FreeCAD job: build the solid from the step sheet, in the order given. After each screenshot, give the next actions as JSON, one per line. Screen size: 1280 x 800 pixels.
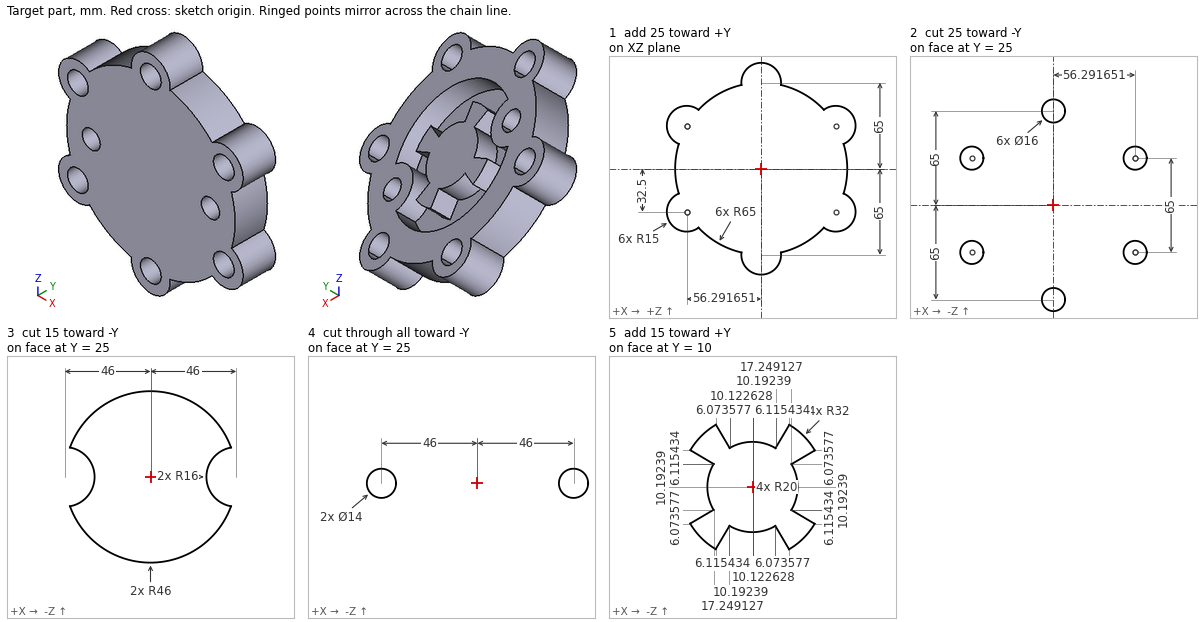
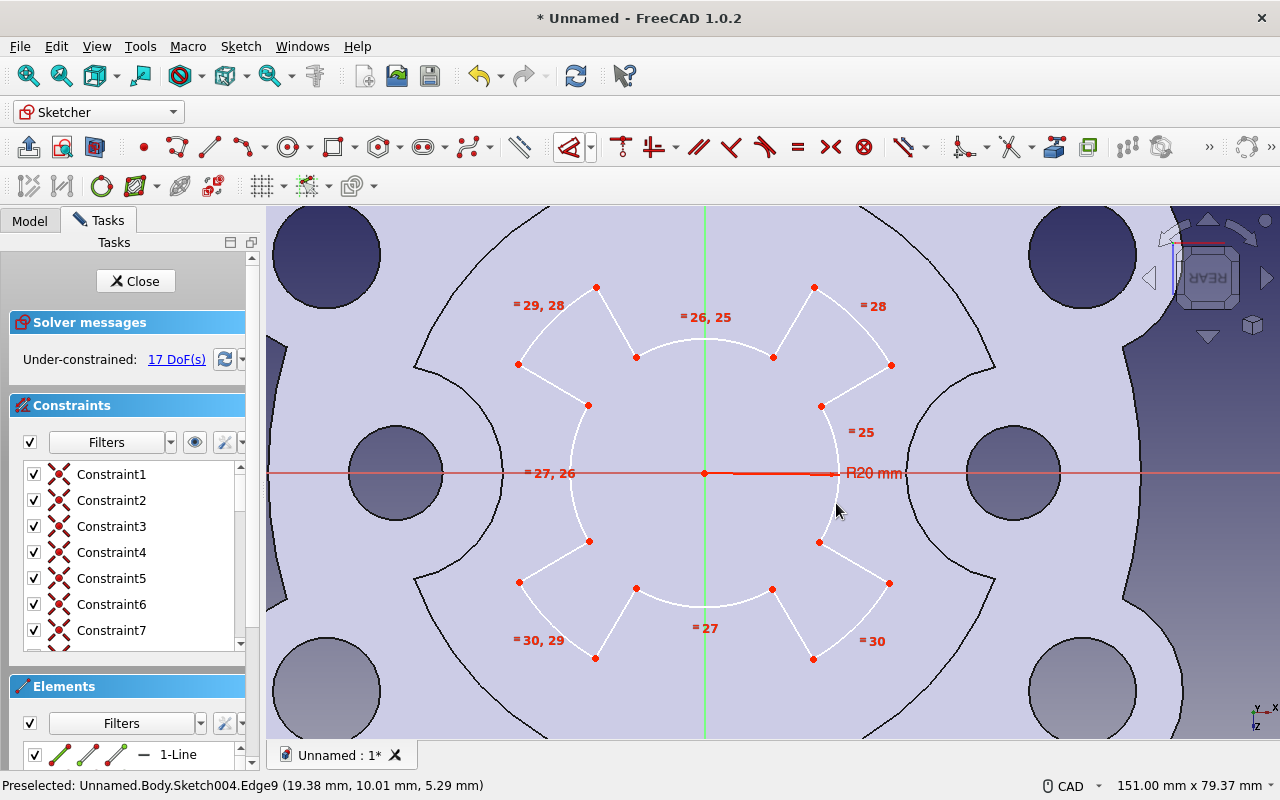
{"action": "left_click", "coordinate": [872, 338]}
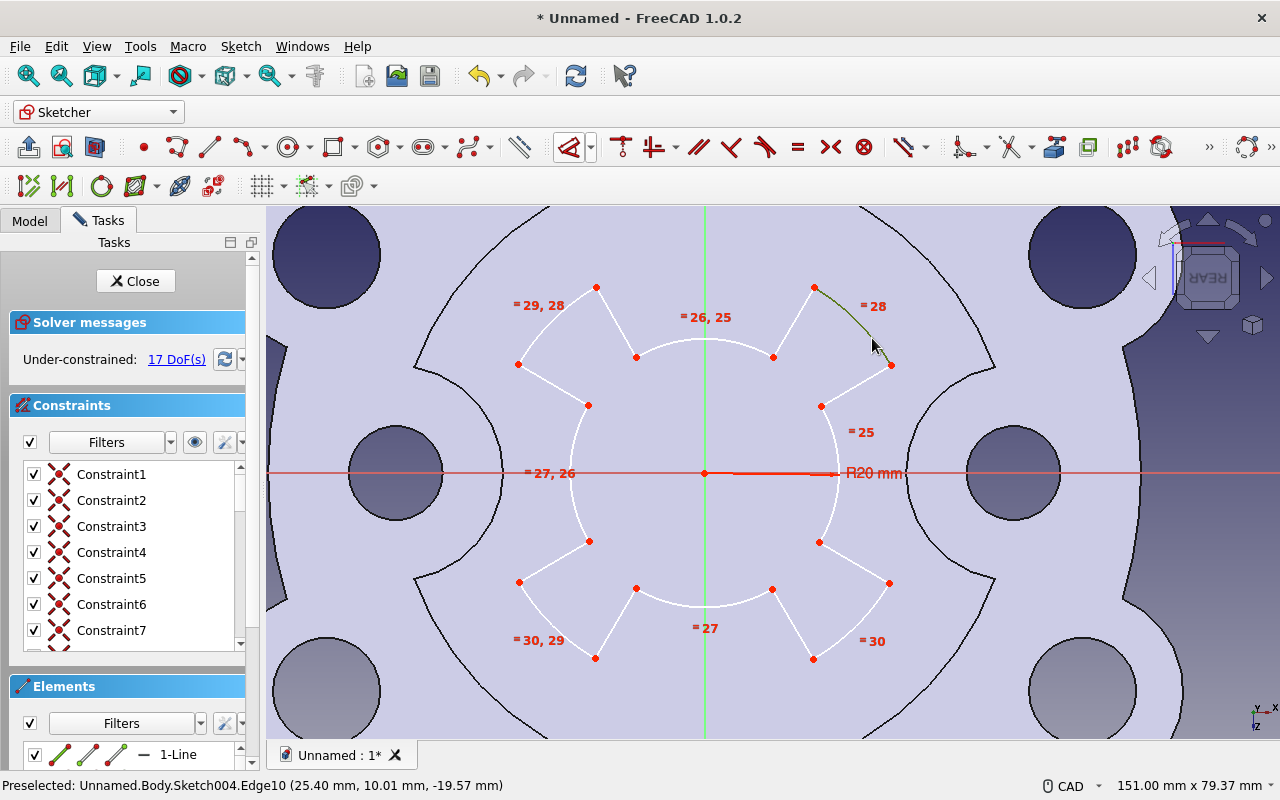
{"action": "left_click", "coordinate": [590, 148]}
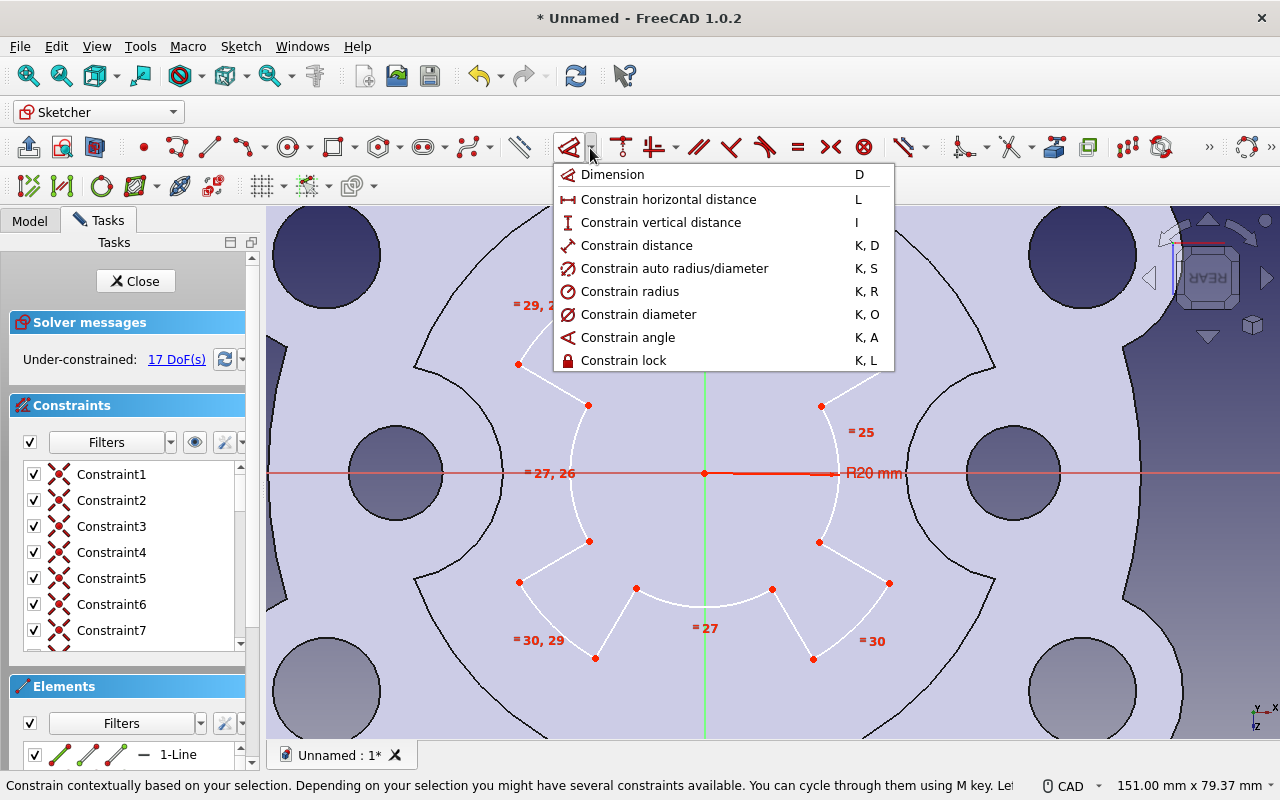
{"action": "left_click", "coordinate": [724, 292]}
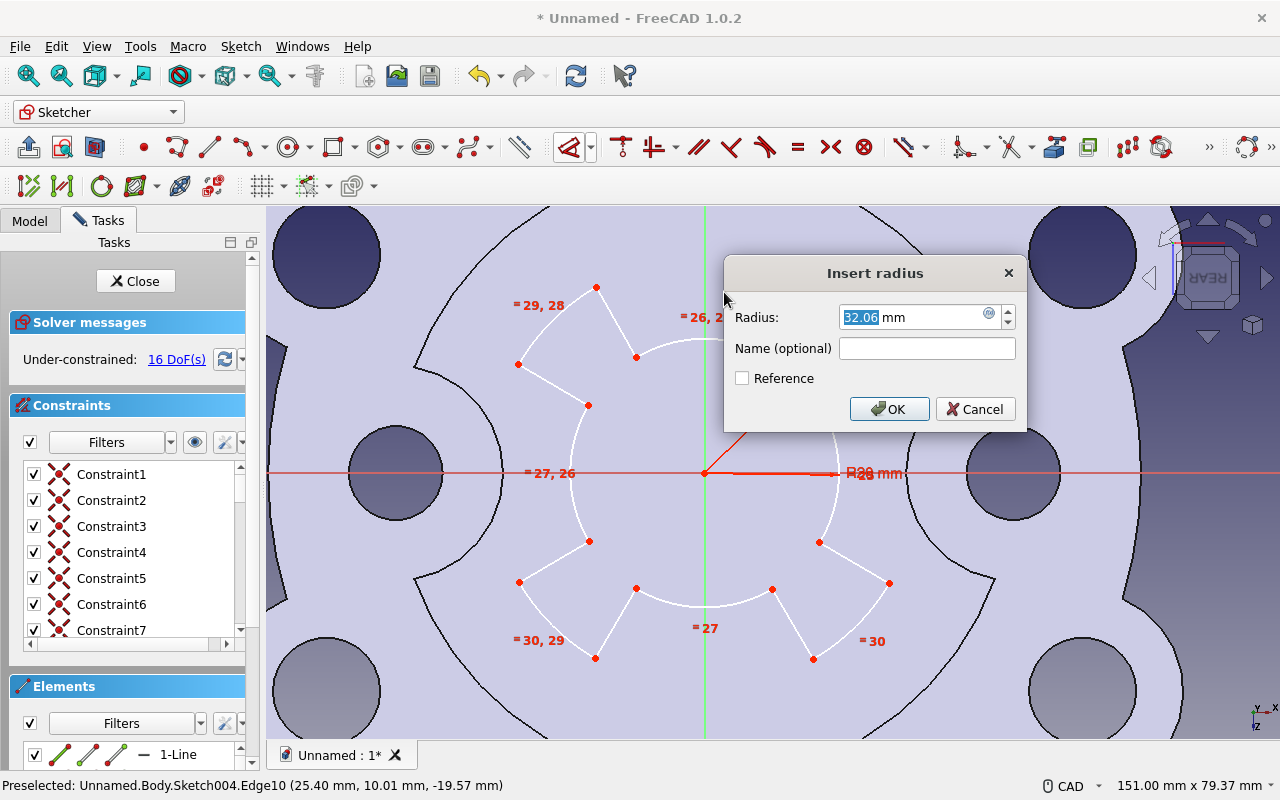
{"action": "type", "text": "32"}
{"action": "key", "text": "Return"}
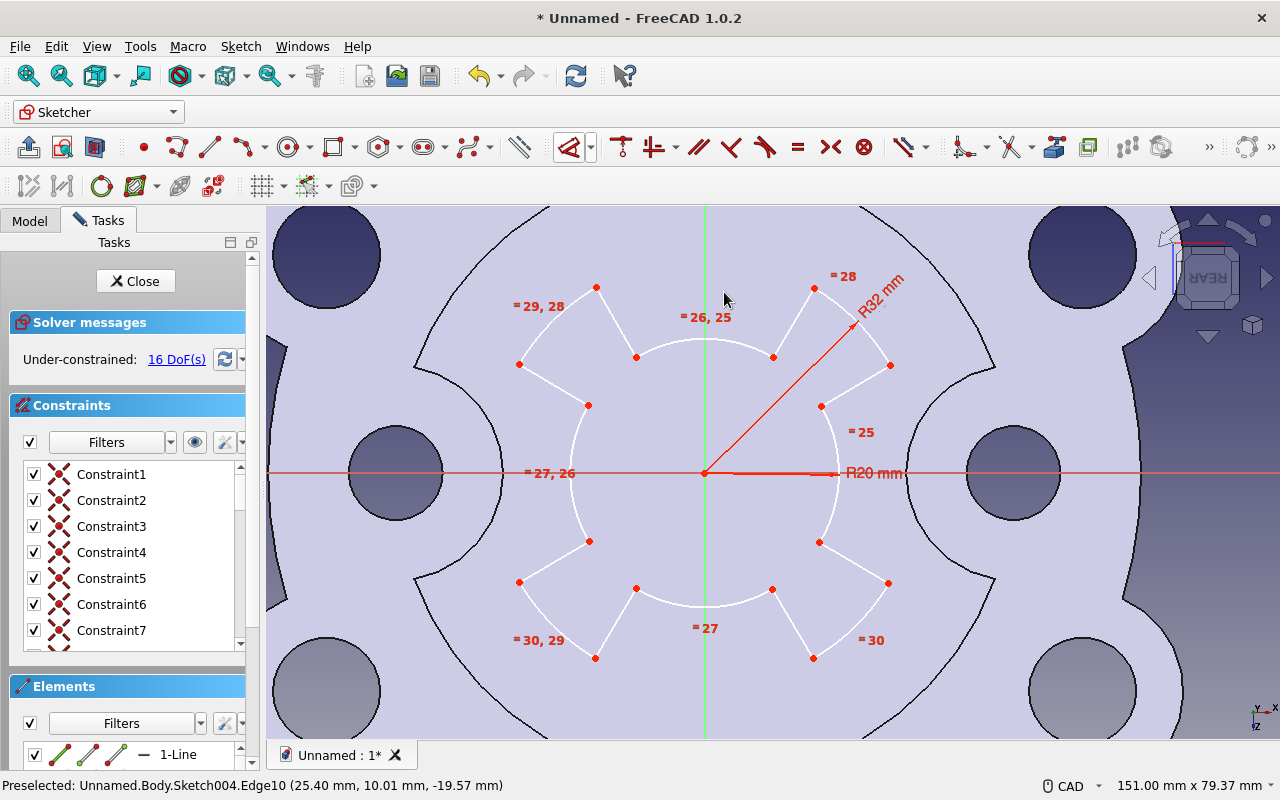
{"action": "left_click", "coordinate": [820, 543]}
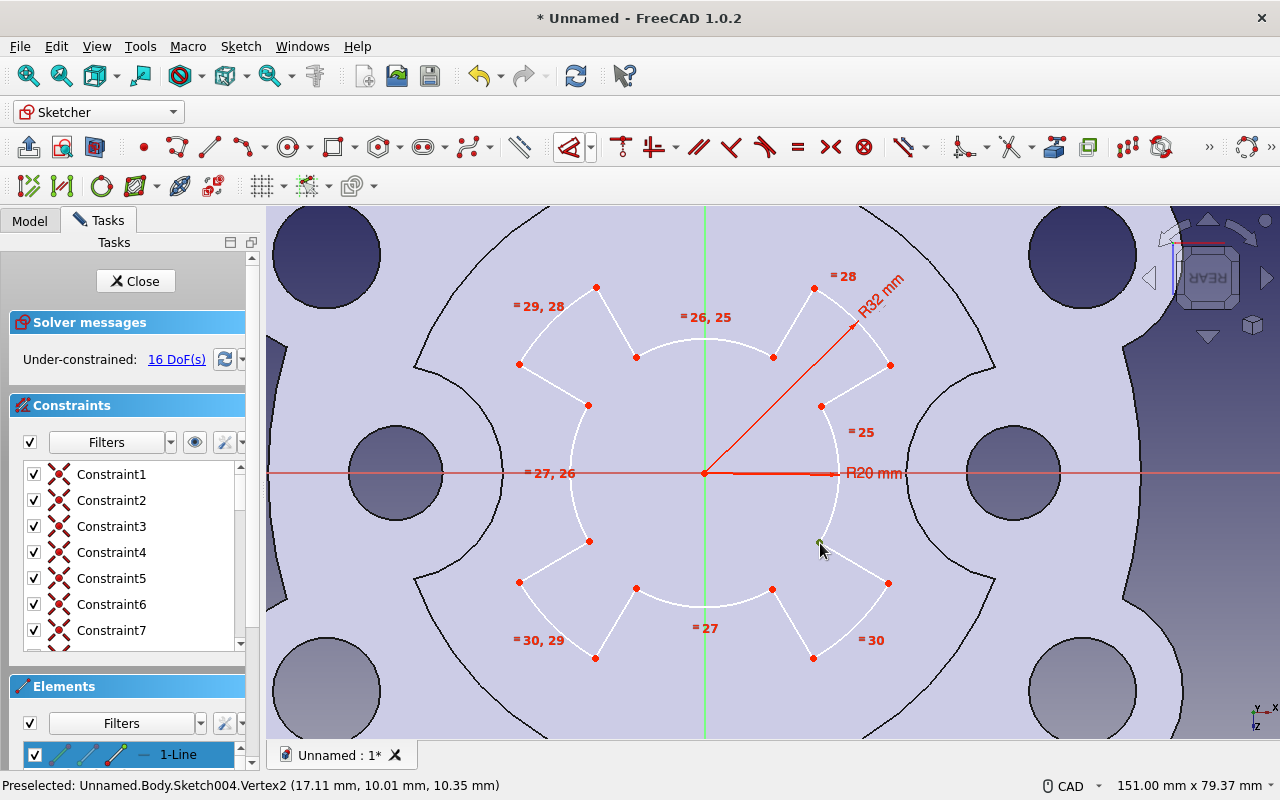
{"action": "key", "text": "i"}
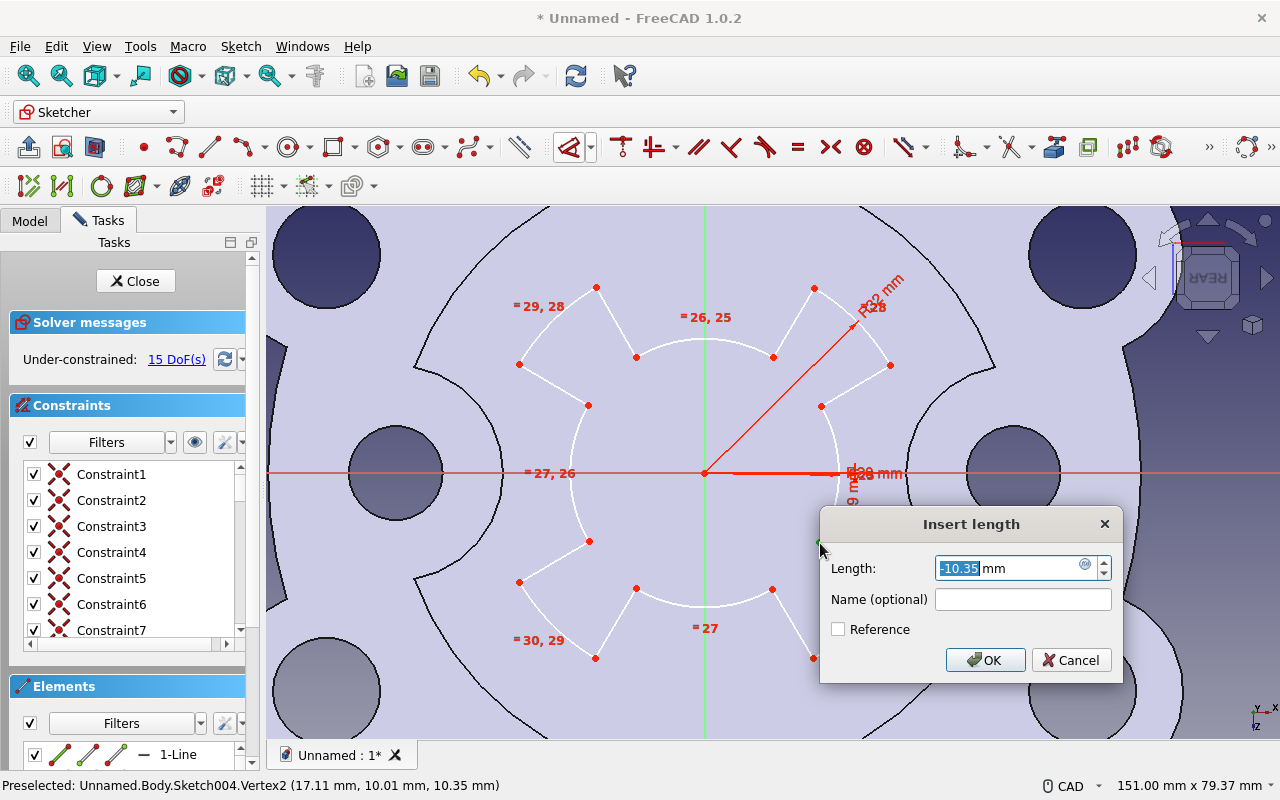
{"action": "type", "text": "-10.19239"}
{"action": "key", "text": "Return"}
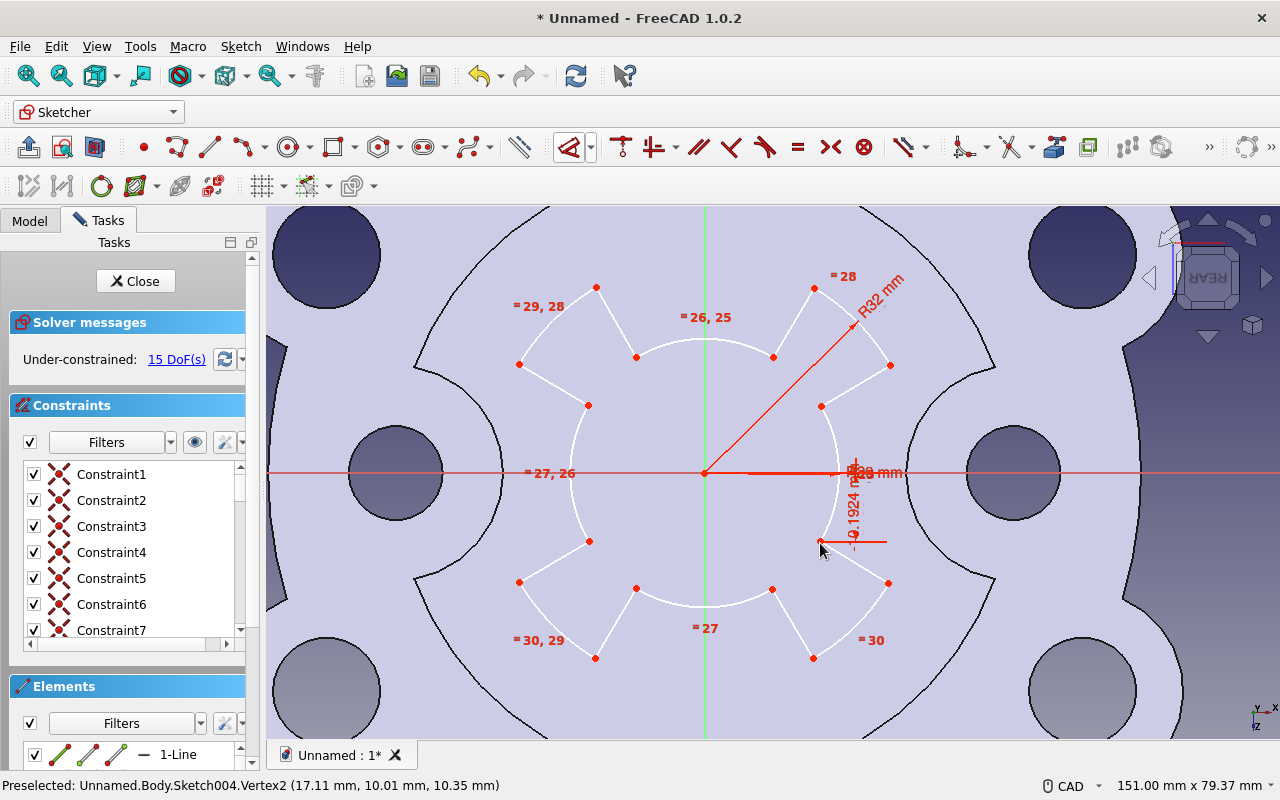
{"action": "left_click", "coordinate": [773, 358]}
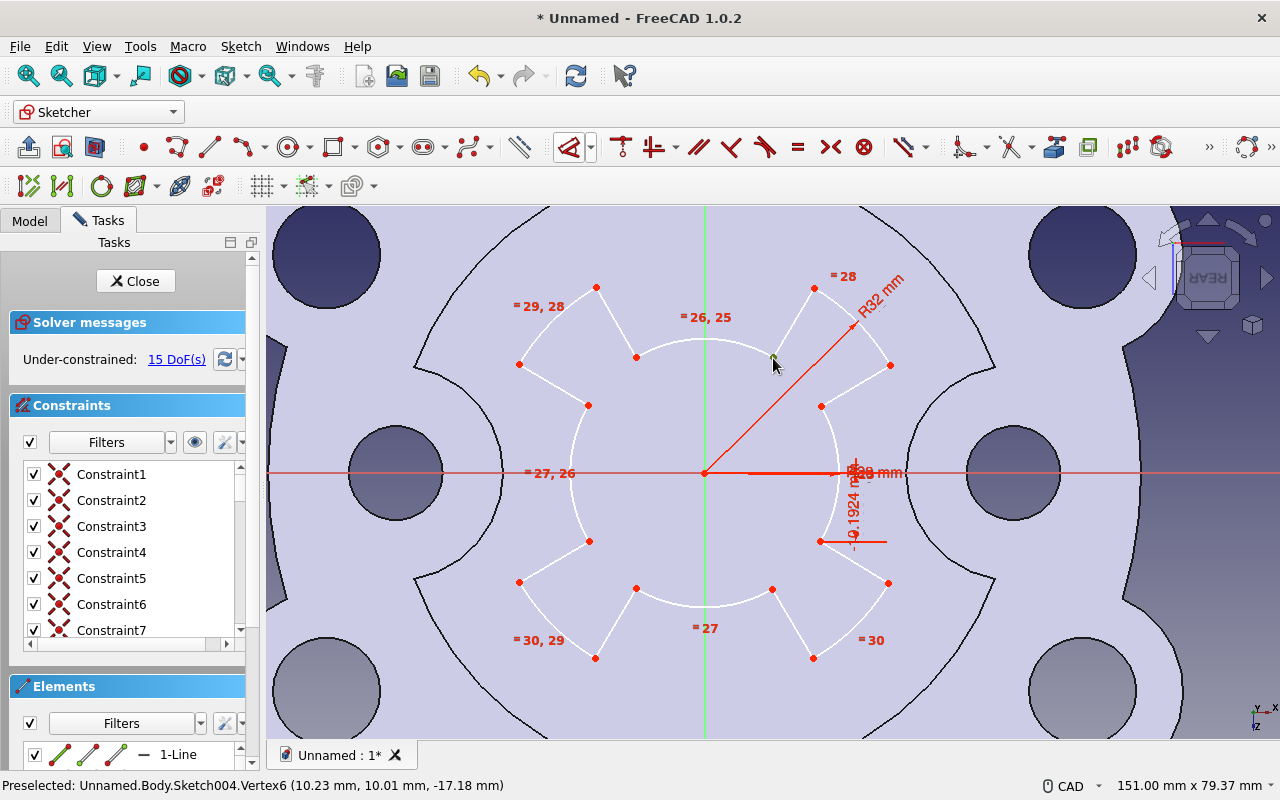
{"action": "key", "text": "l"}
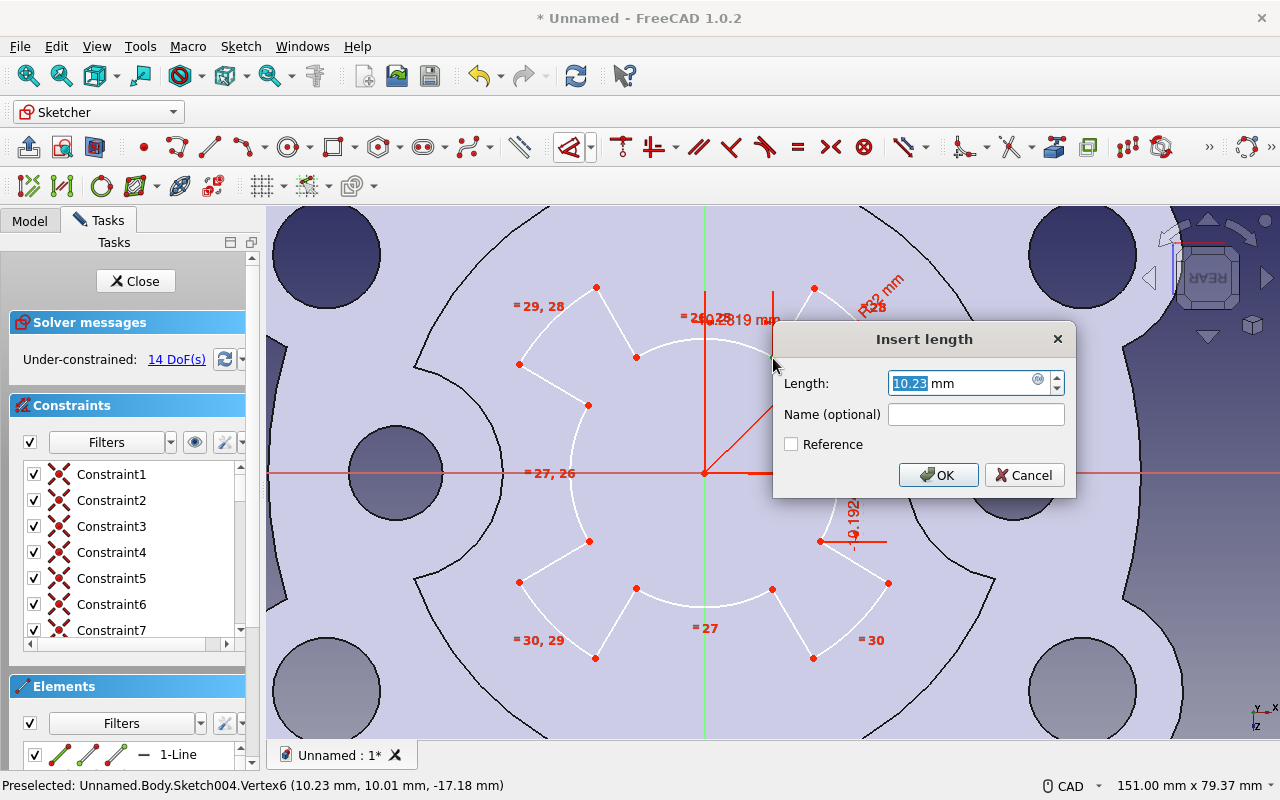
{"action": "type", "text": "10.19239"}
{"action": "key", "text": "Return"}